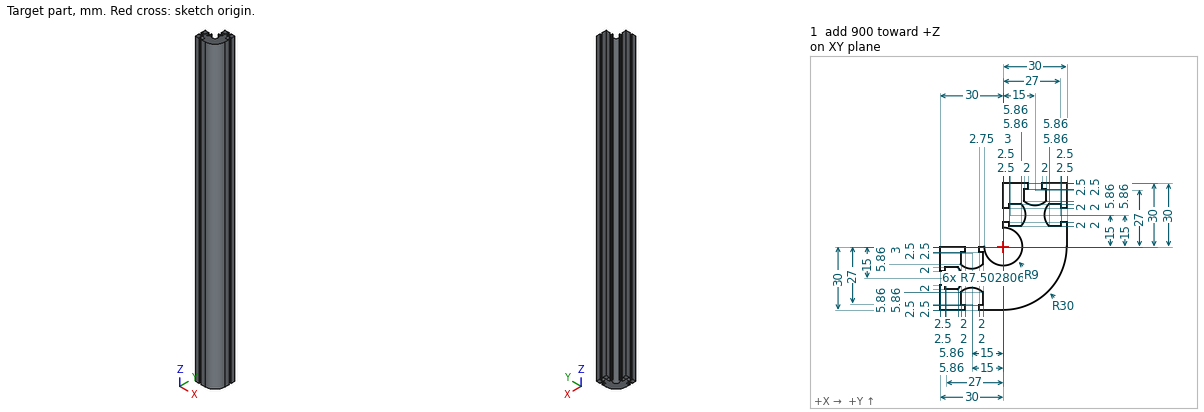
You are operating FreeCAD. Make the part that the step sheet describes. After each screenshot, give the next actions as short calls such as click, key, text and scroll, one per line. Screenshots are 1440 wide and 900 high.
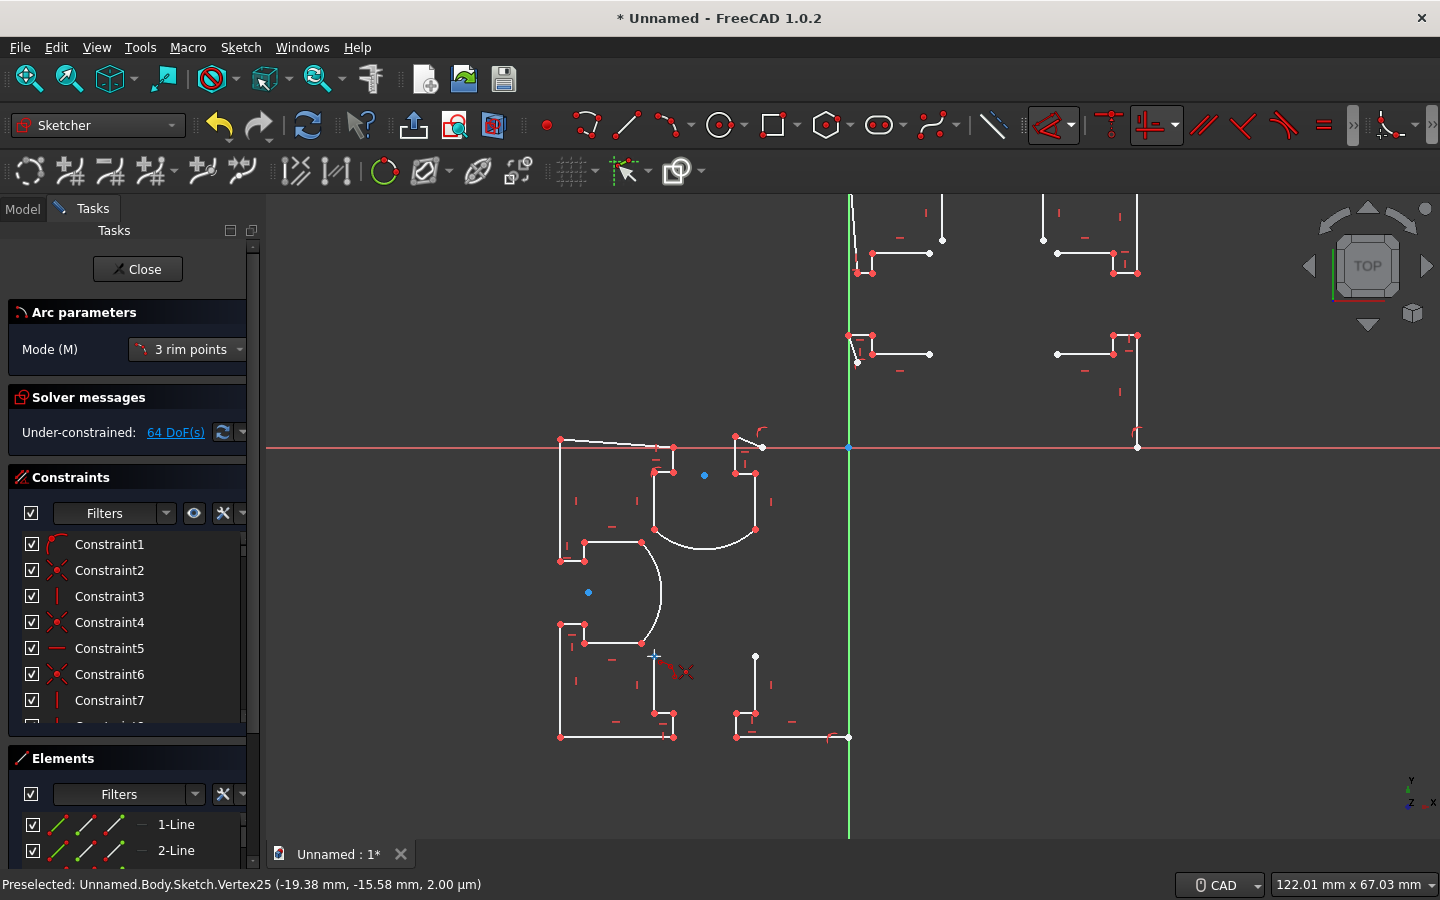
click(654, 656)
click(755, 656)
click(704, 635)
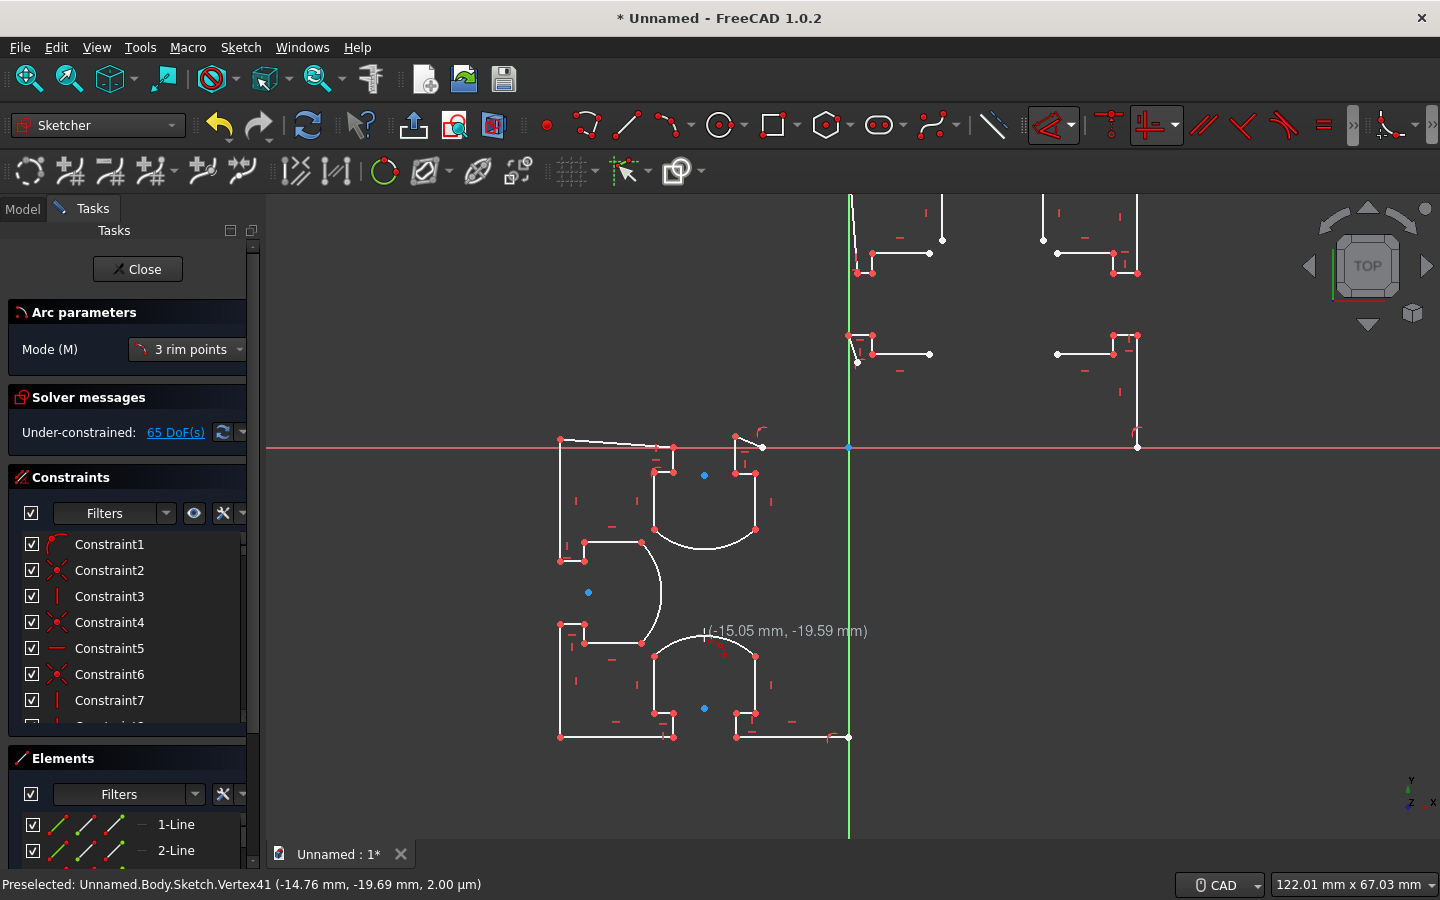
click(849, 737)
click(1137, 448)
click(1053, 652)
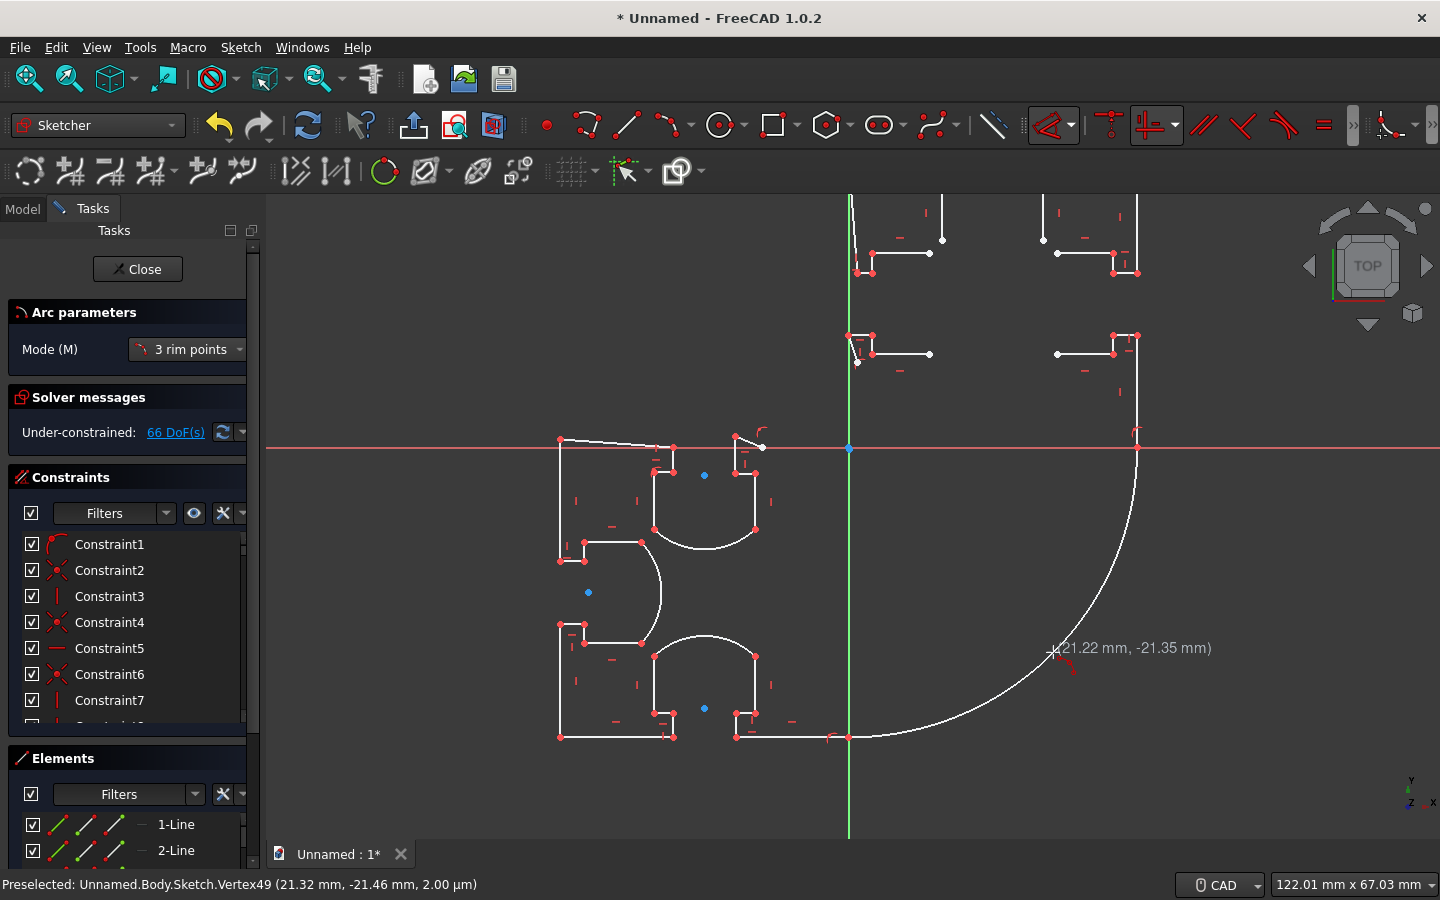
click(1057, 354)
click(1057, 253)
click(1036, 303)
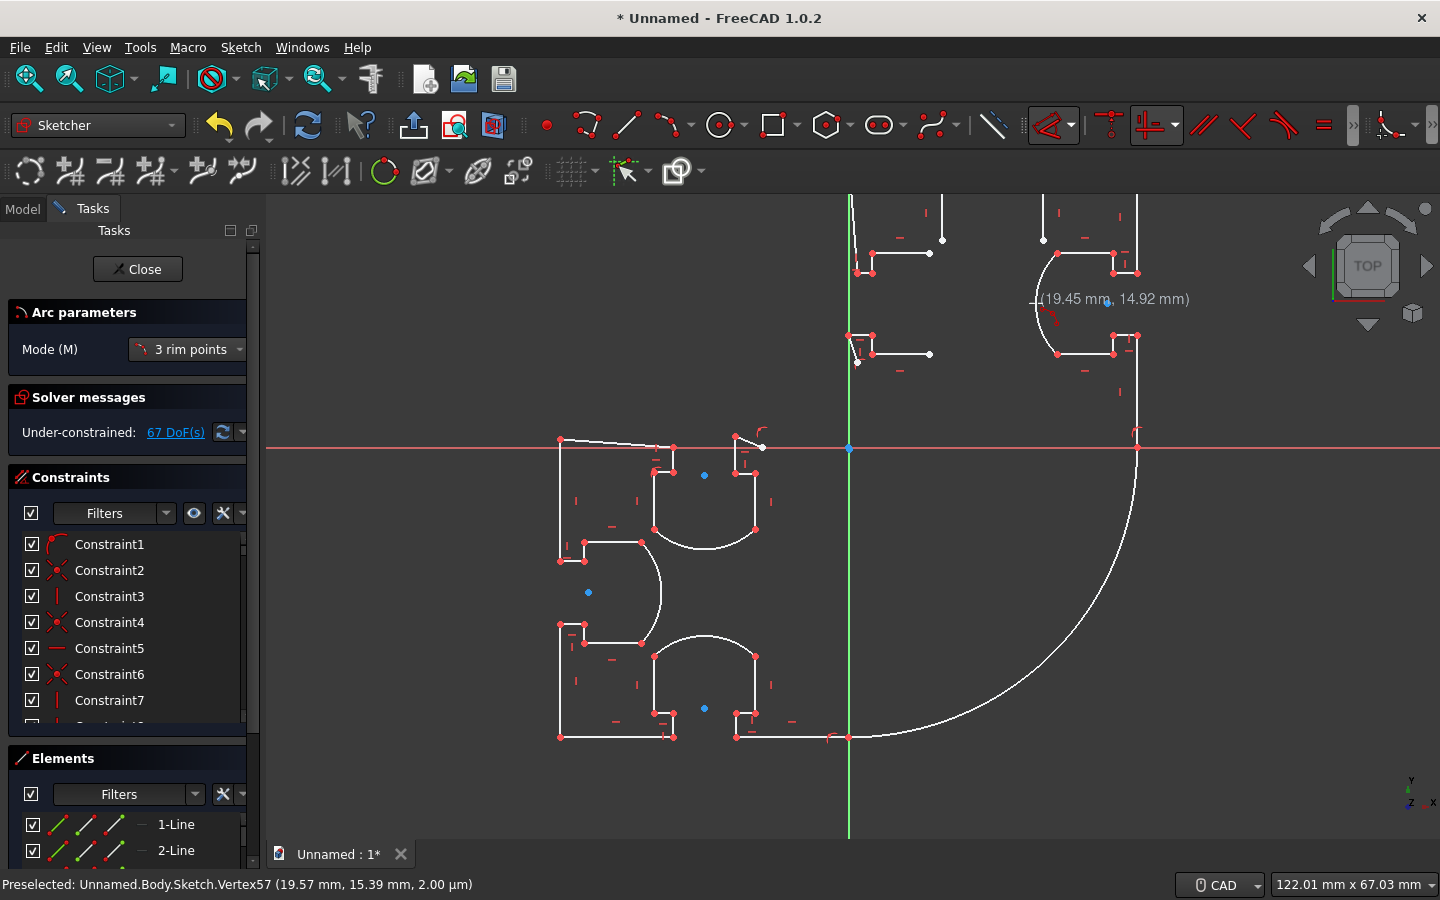
click(1043, 240)
click(942, 240)
click(993, 260)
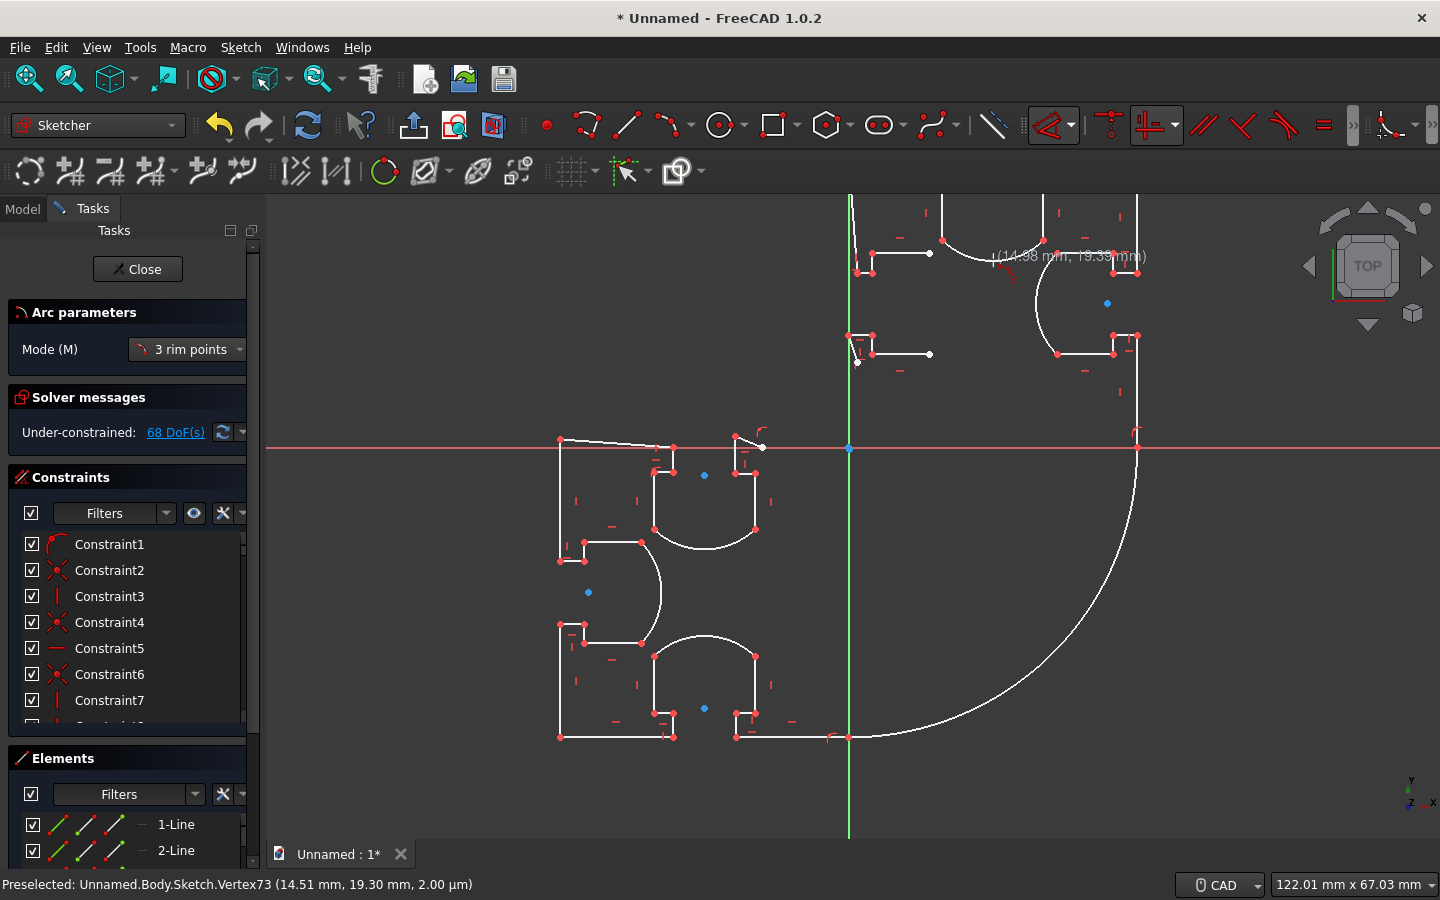
click(929, 253)
click(929, 354)
click(950, 303)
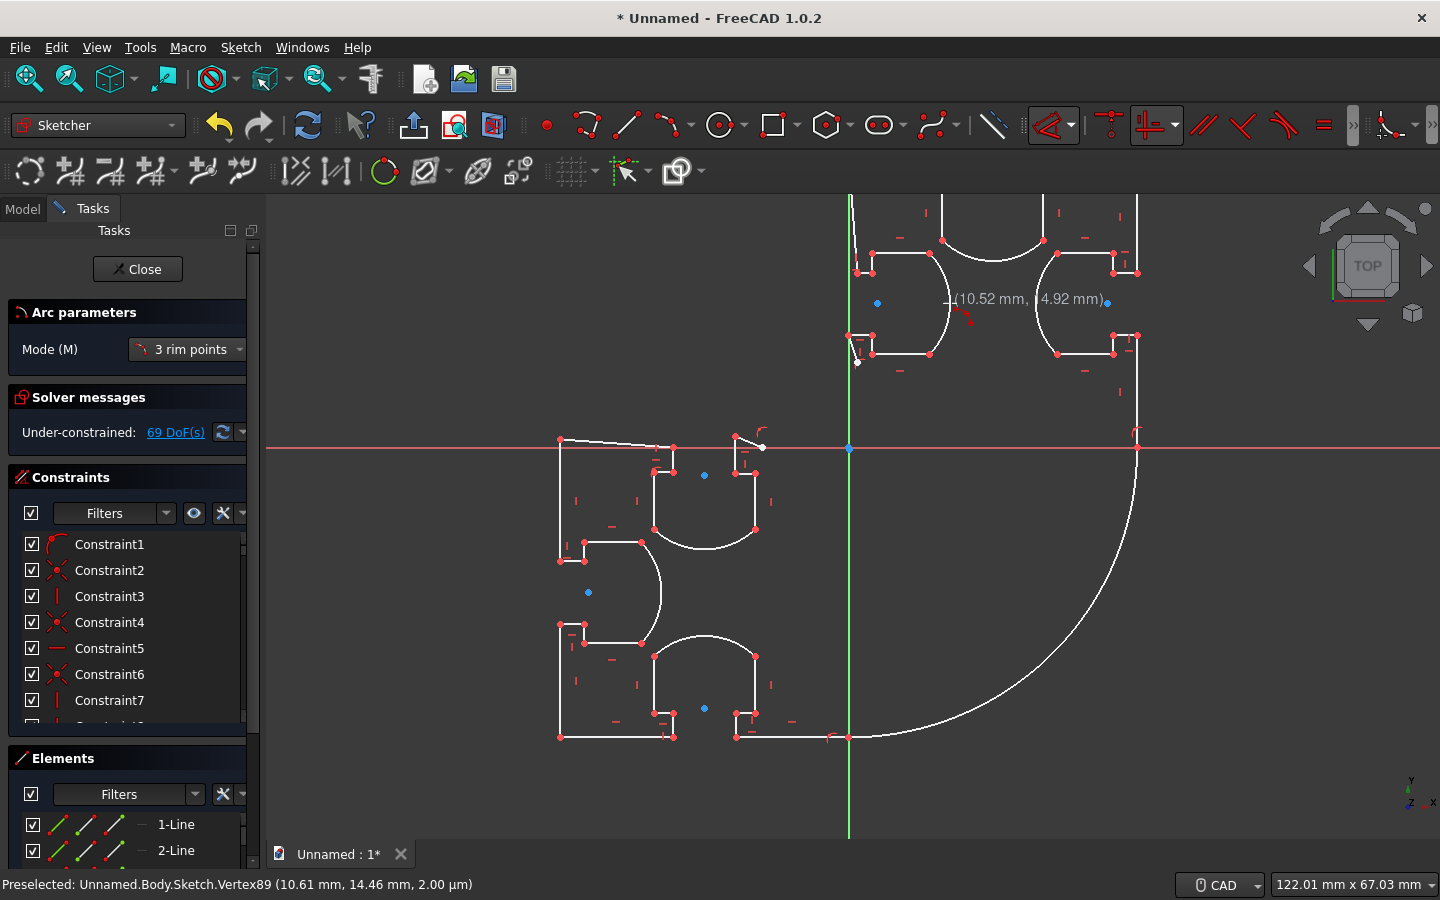
click(857, 362)
click(762, 448)
click(910, 509)
key(Escape)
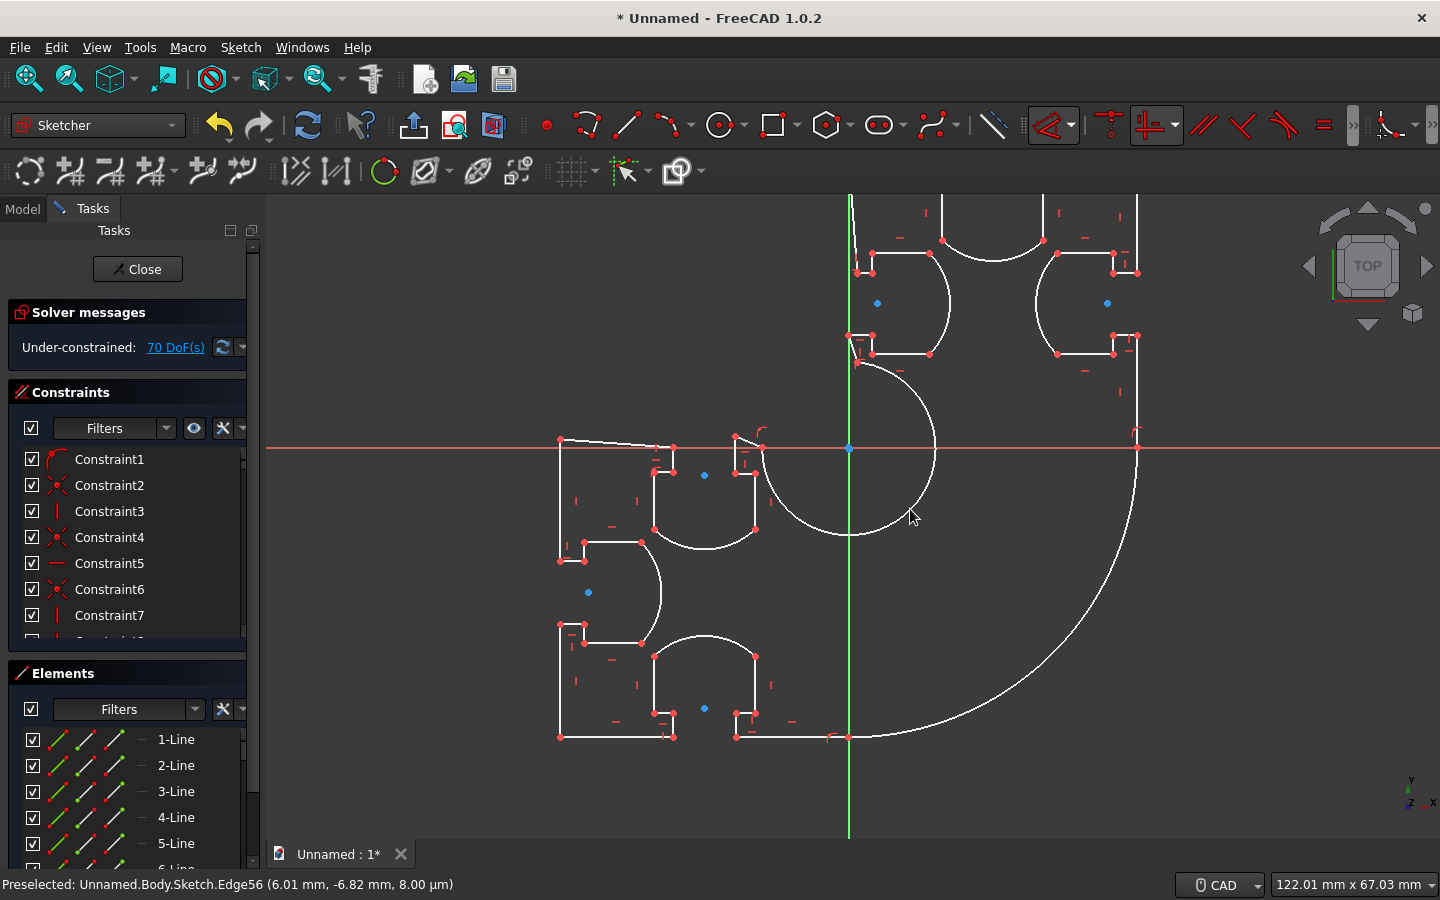
scroll(754, 444, up, 3)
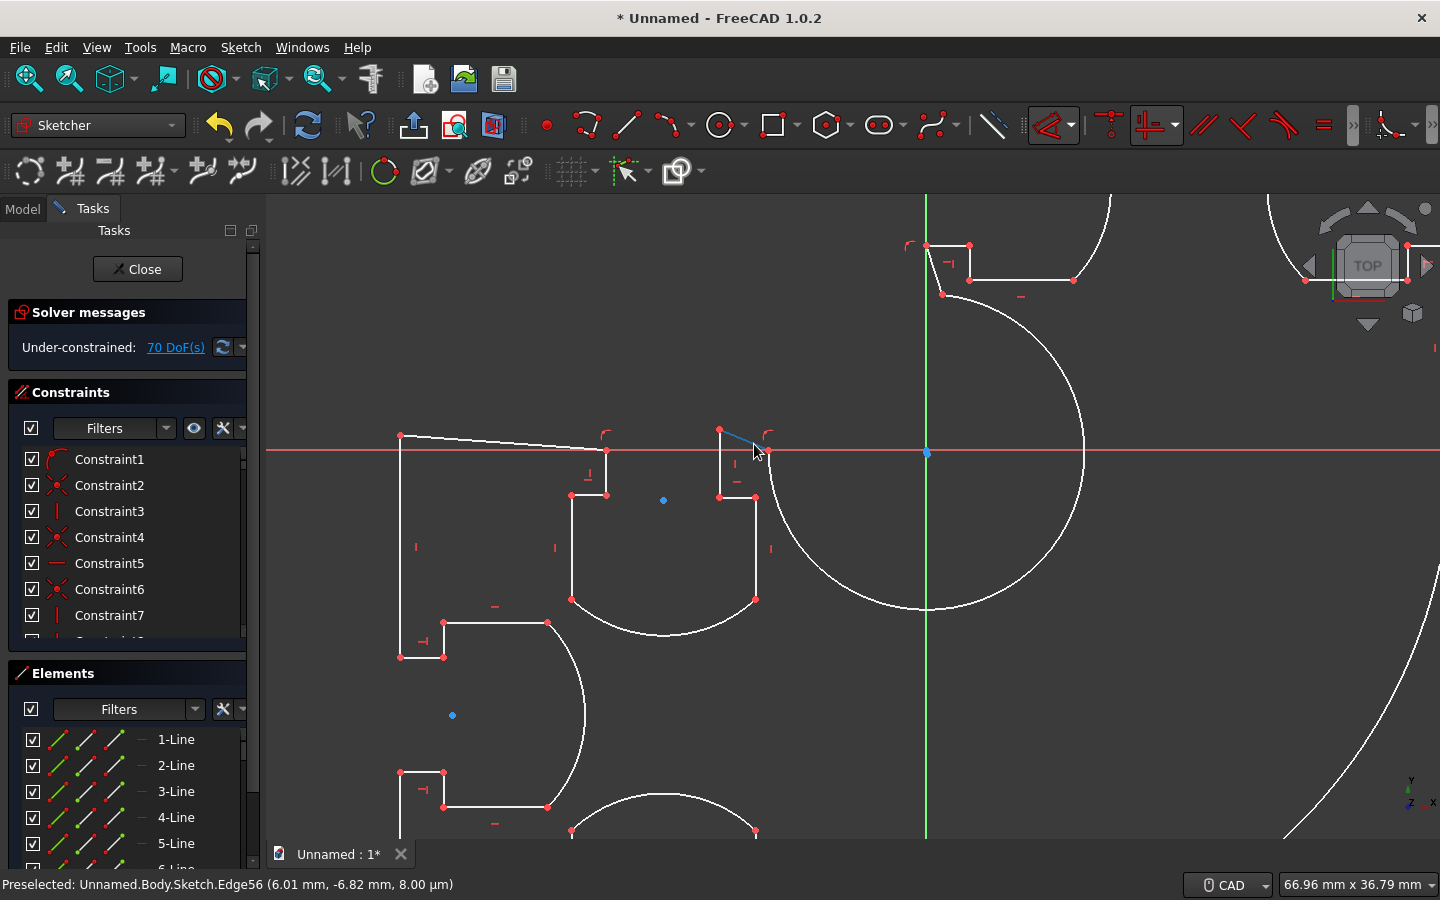
click(754, 444)